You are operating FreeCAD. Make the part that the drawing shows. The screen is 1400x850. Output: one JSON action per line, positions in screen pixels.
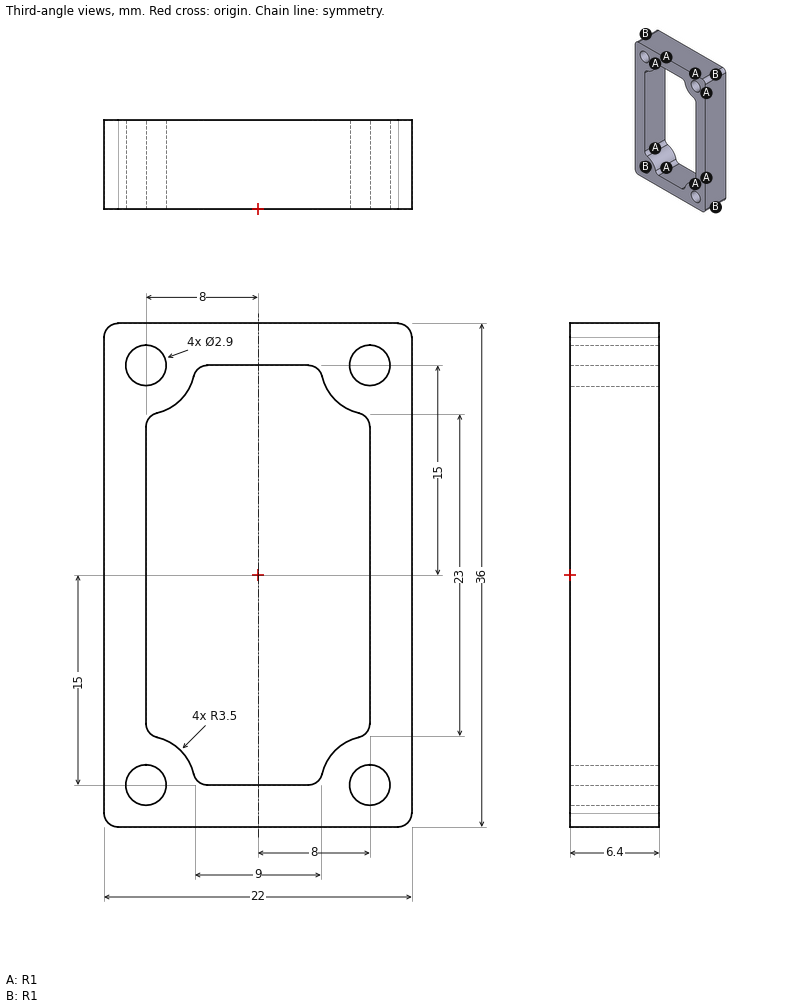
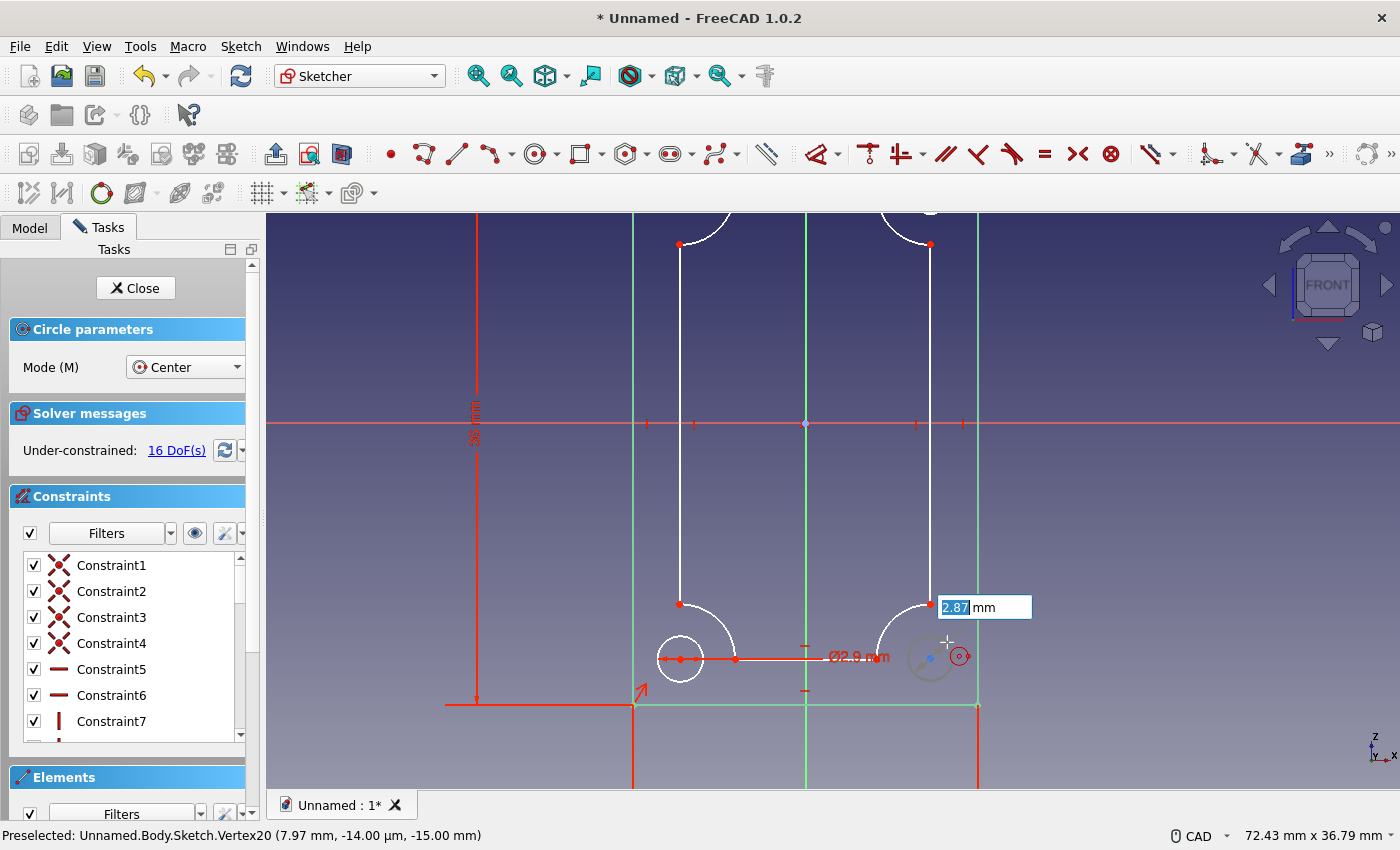
{"action": "type", "text": "2.9"}
{"action": "key", "text": "Return"}
{"action": "key", "text": "Escape"}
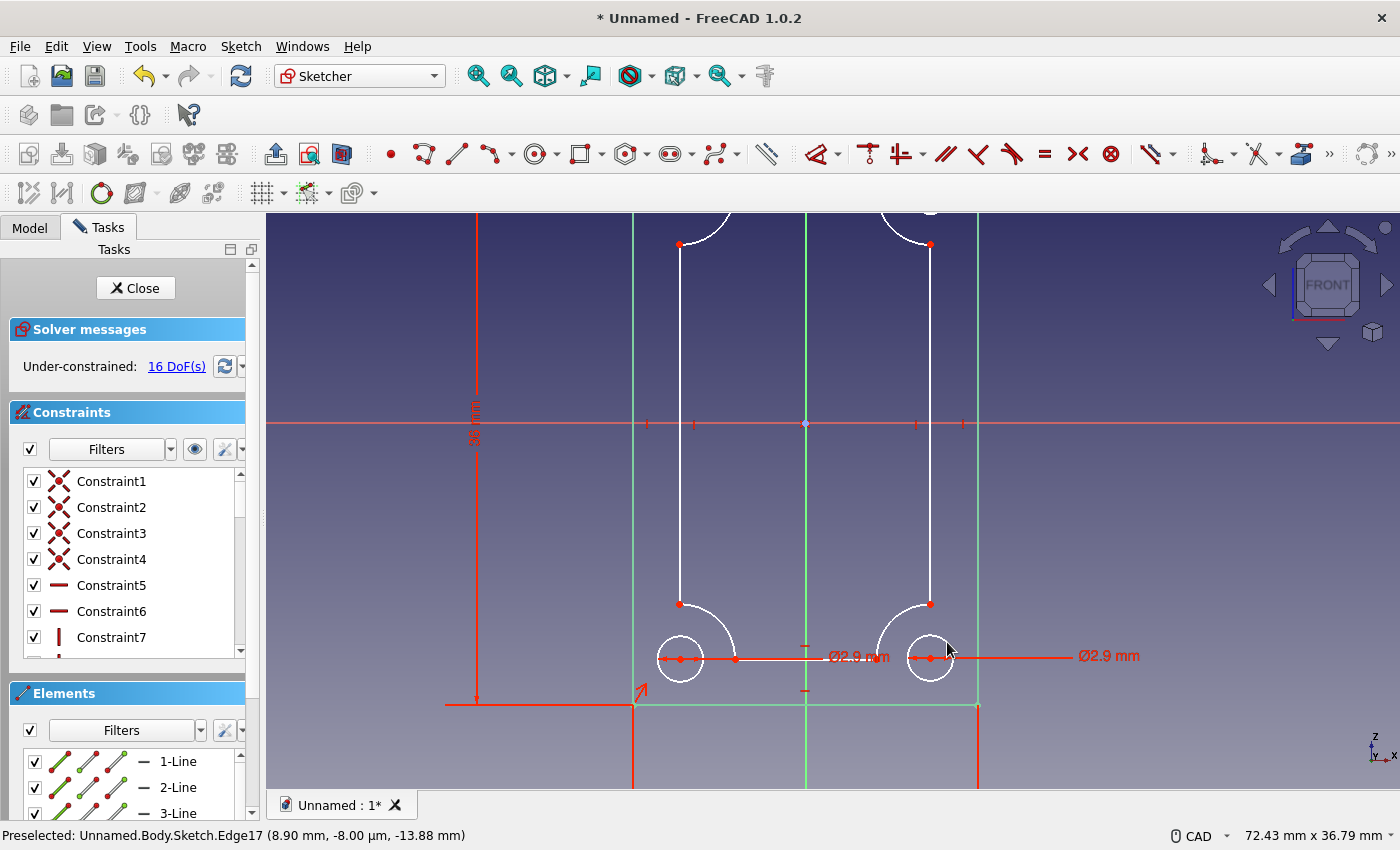
{"action": "left_click", "coordinate": [906, 610]}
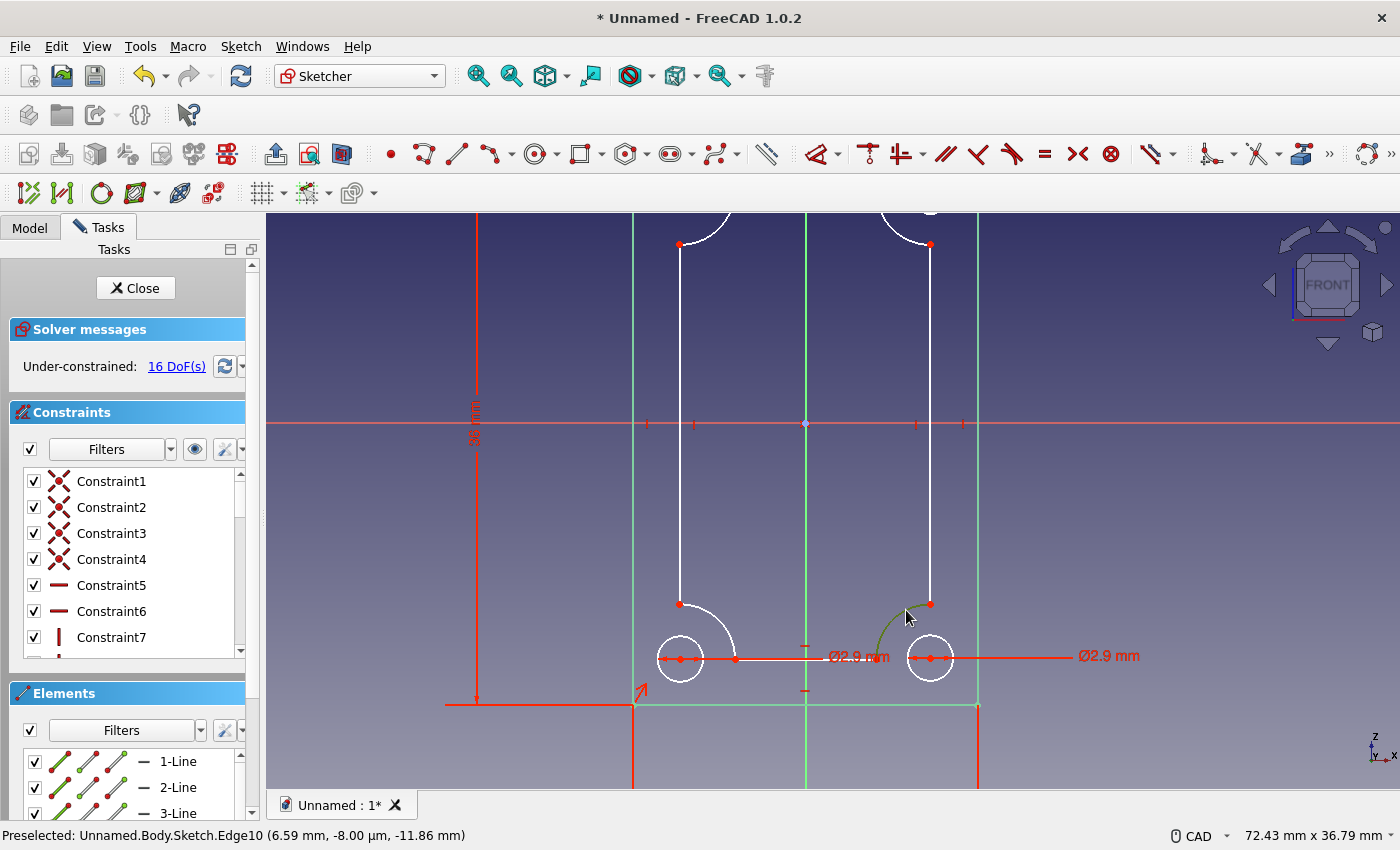
{"action": "left_click", "coordinate": [914, 242]}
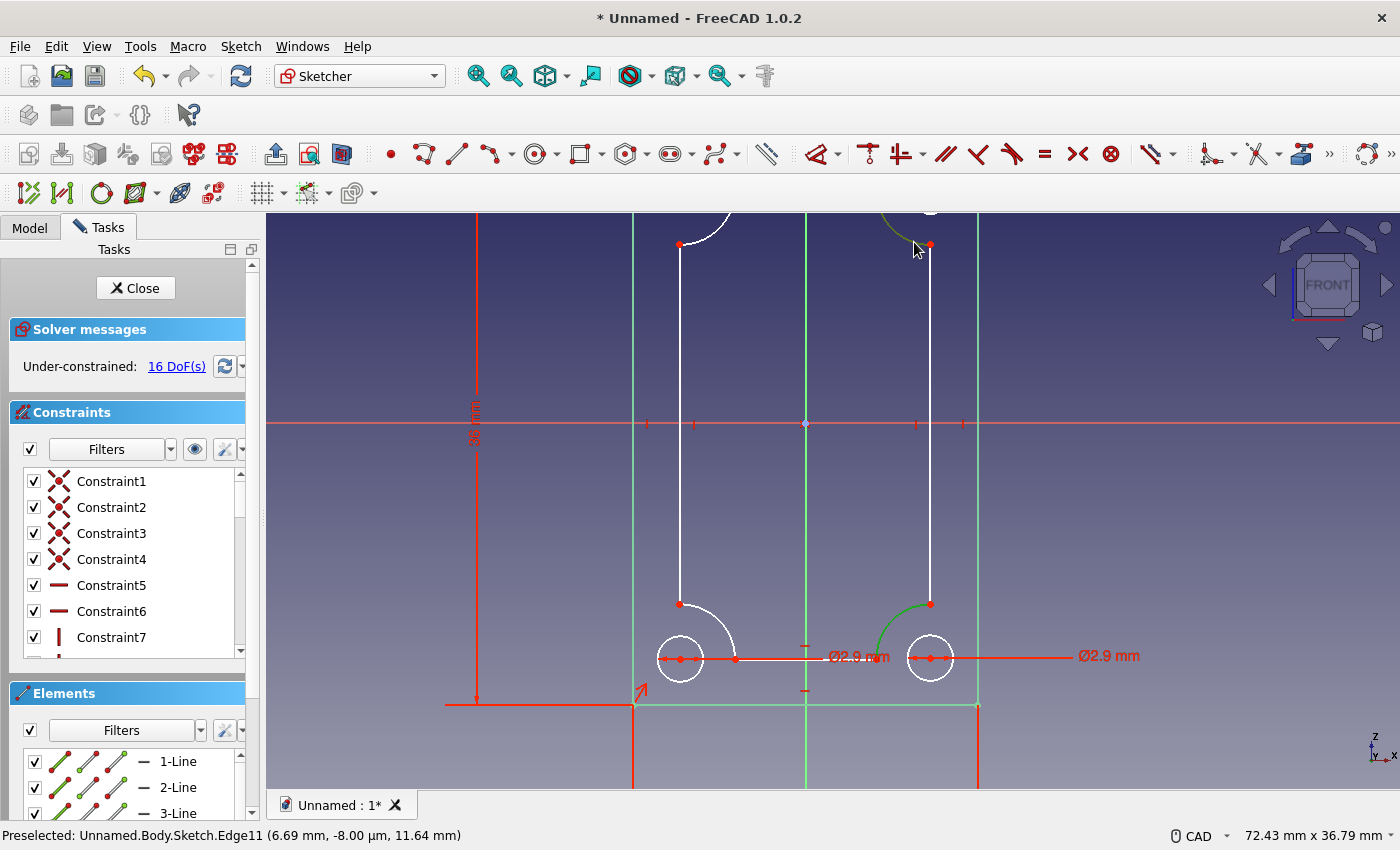
{"action": "left_click", "coordinate": [697, 242]}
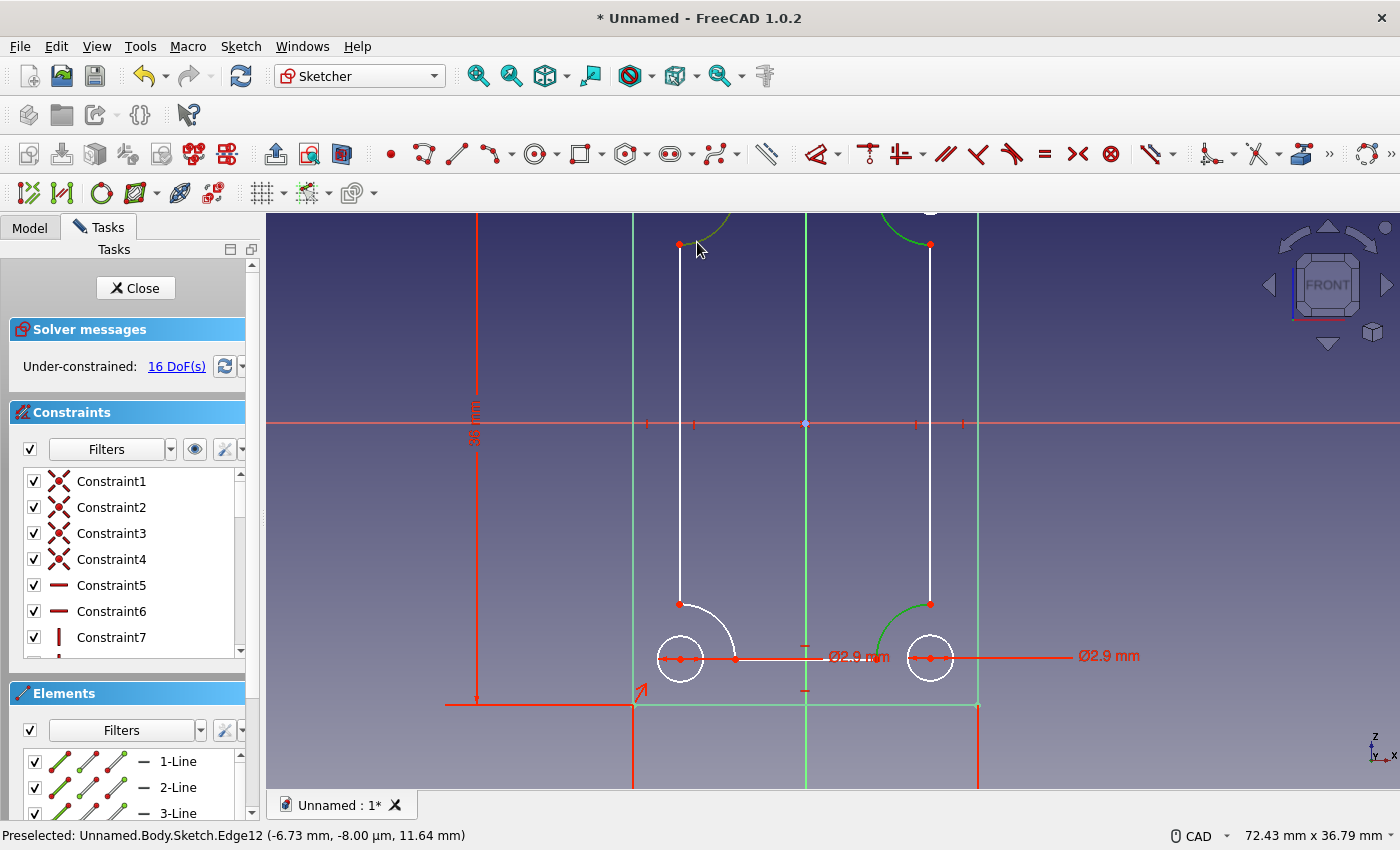
{"action": "left_click", "coordinate": [729, 634]}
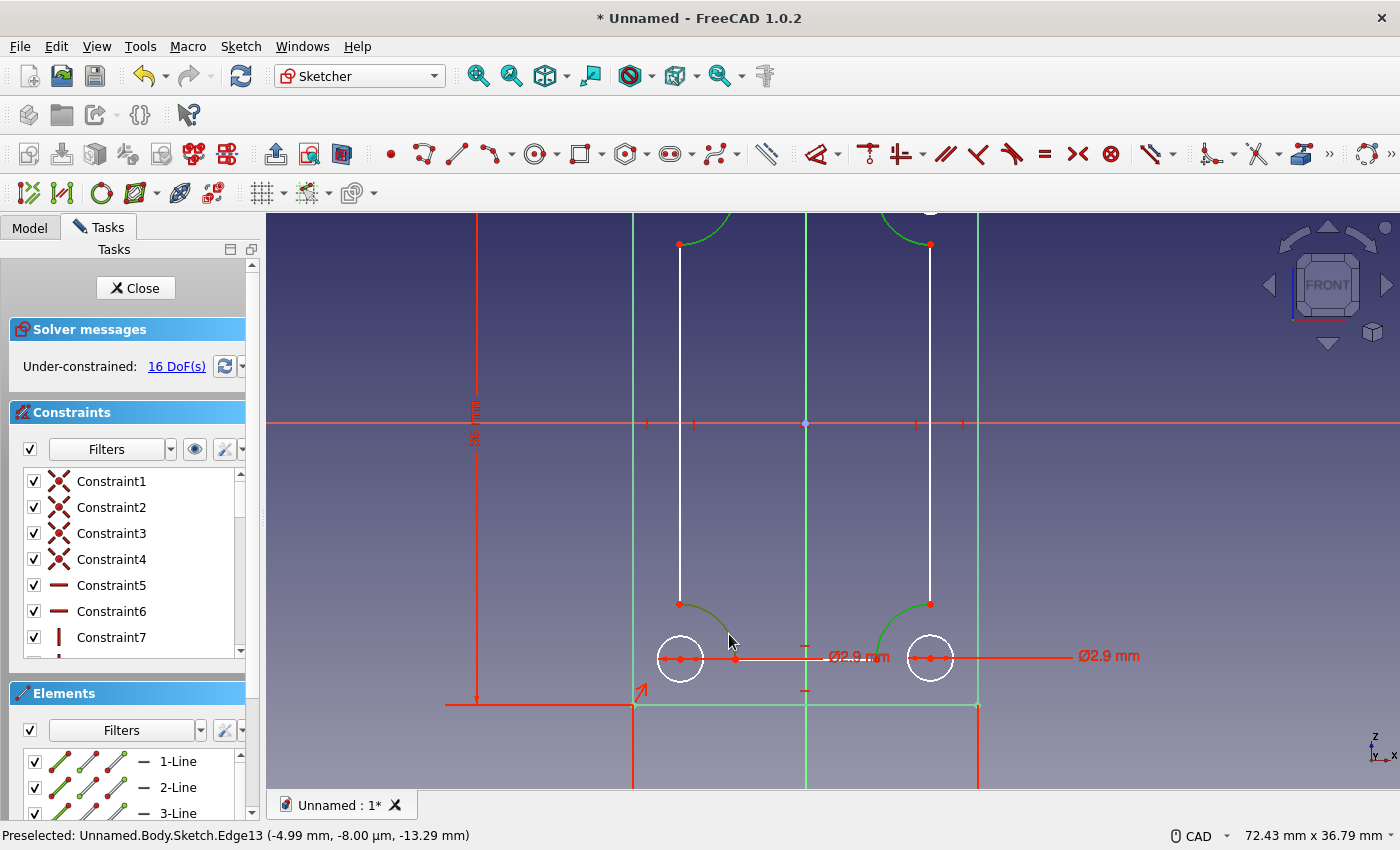
{"action": "left_click", "coordinate": [1045, 154]}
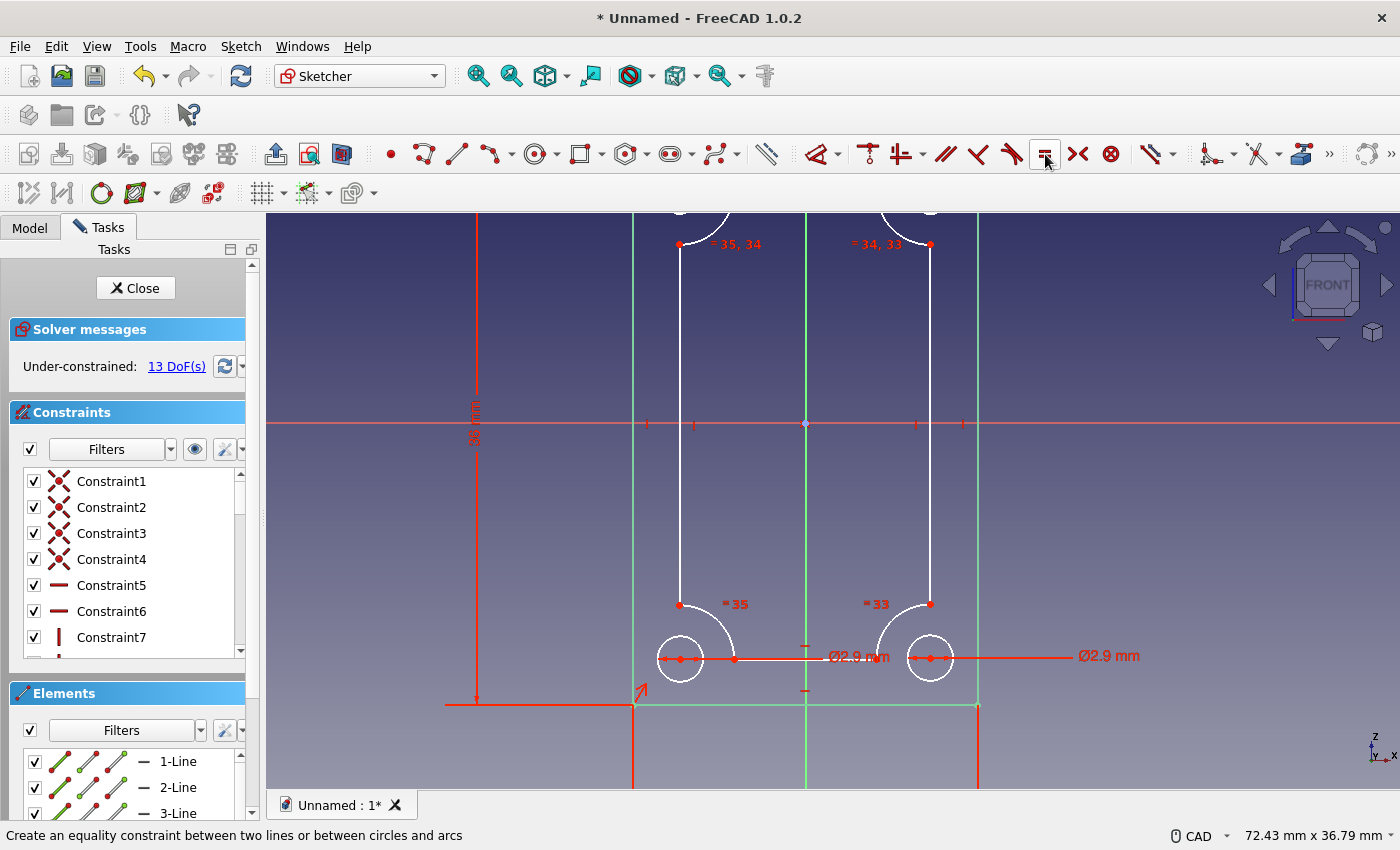
{"action": "left_click", "coordinate": [930, 658]}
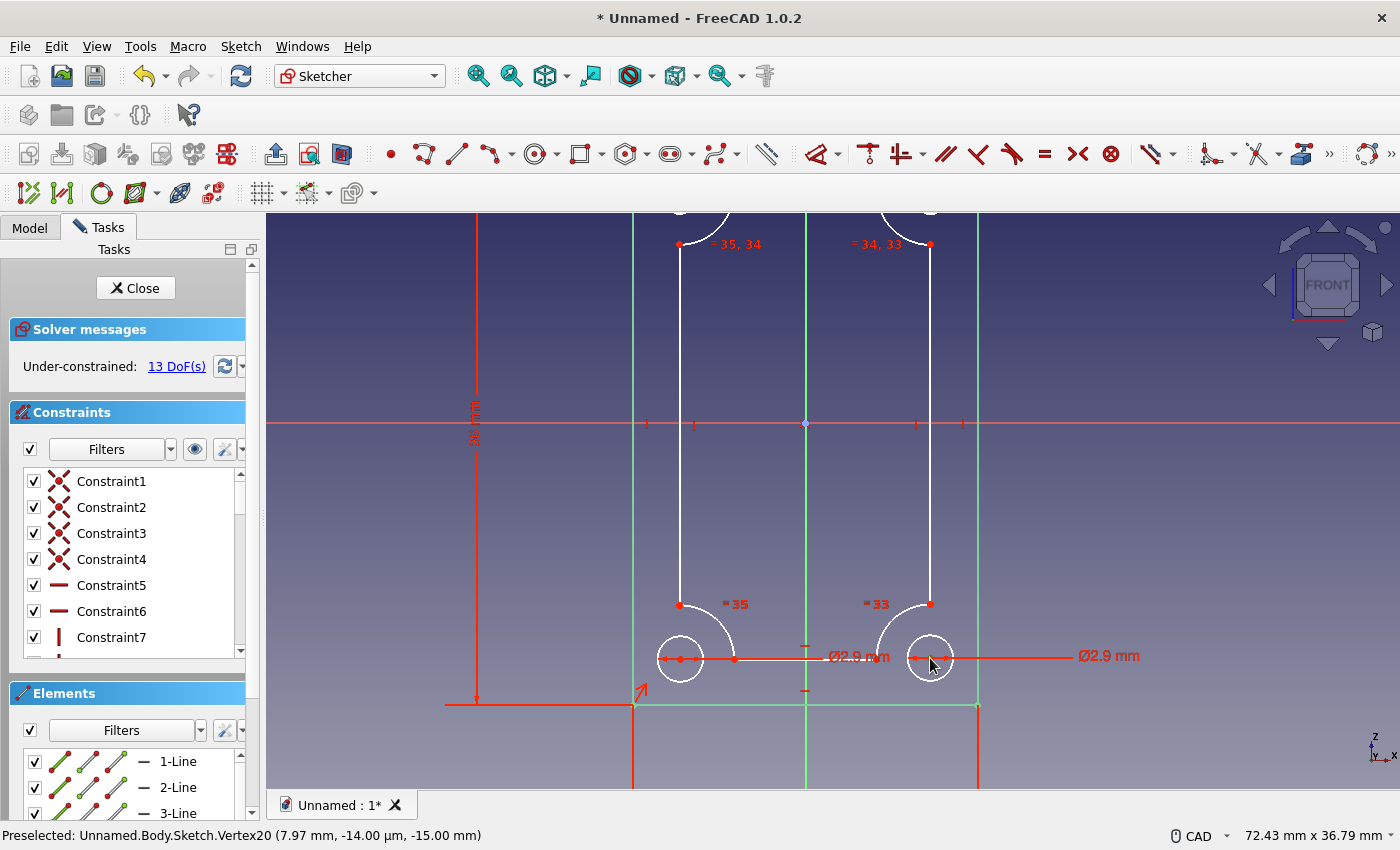
{"action": "scroll", "coordinate": [681, 659], "scroll_direction": "down", "scroll_amount": 2}